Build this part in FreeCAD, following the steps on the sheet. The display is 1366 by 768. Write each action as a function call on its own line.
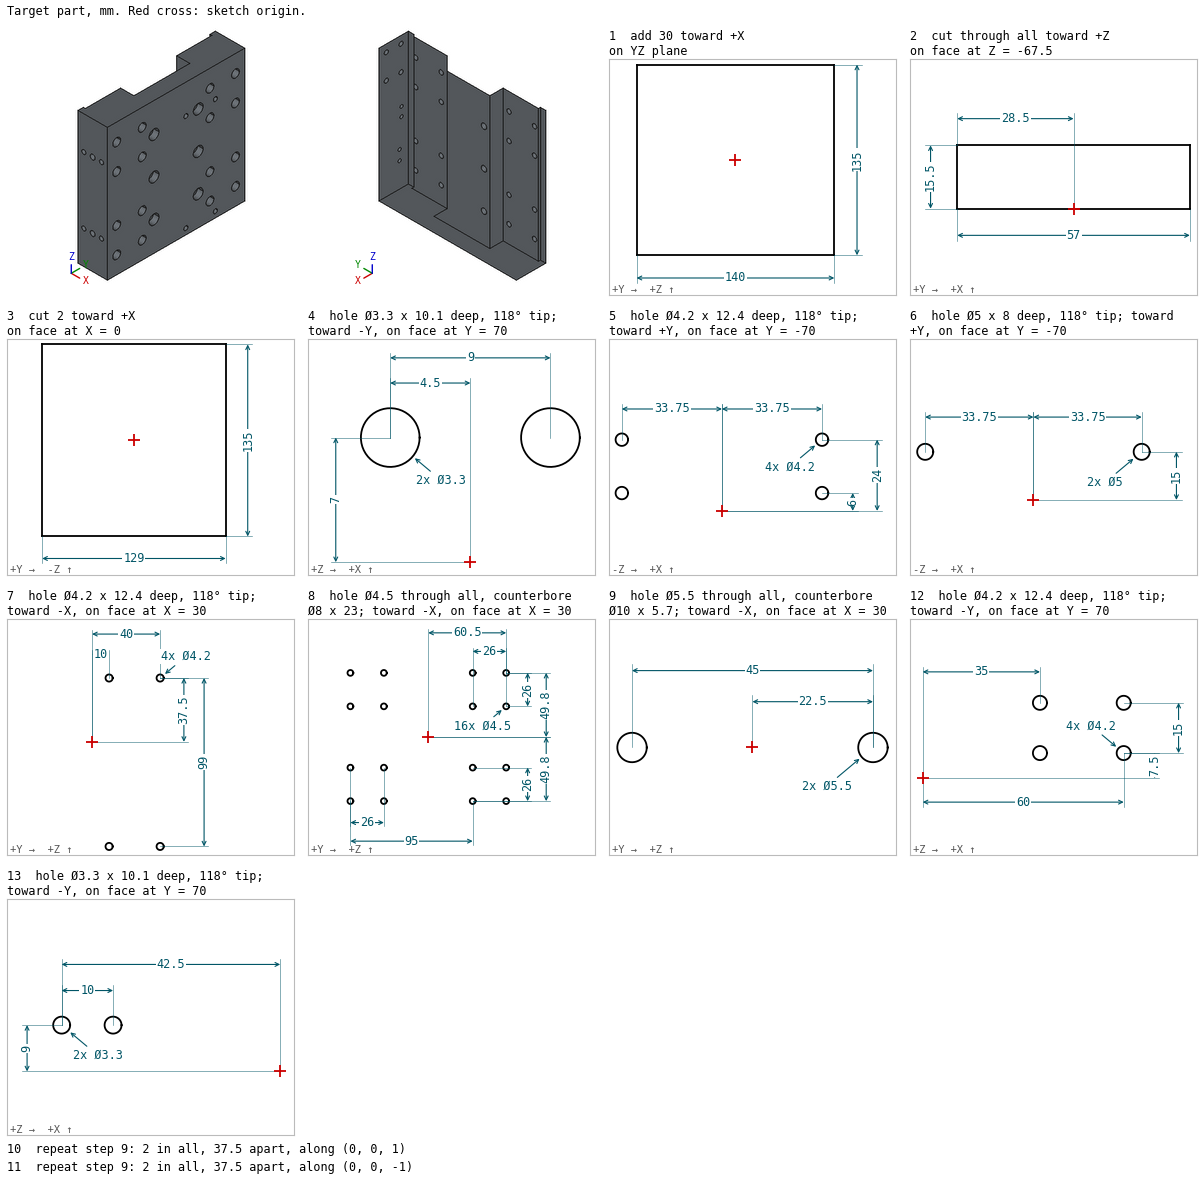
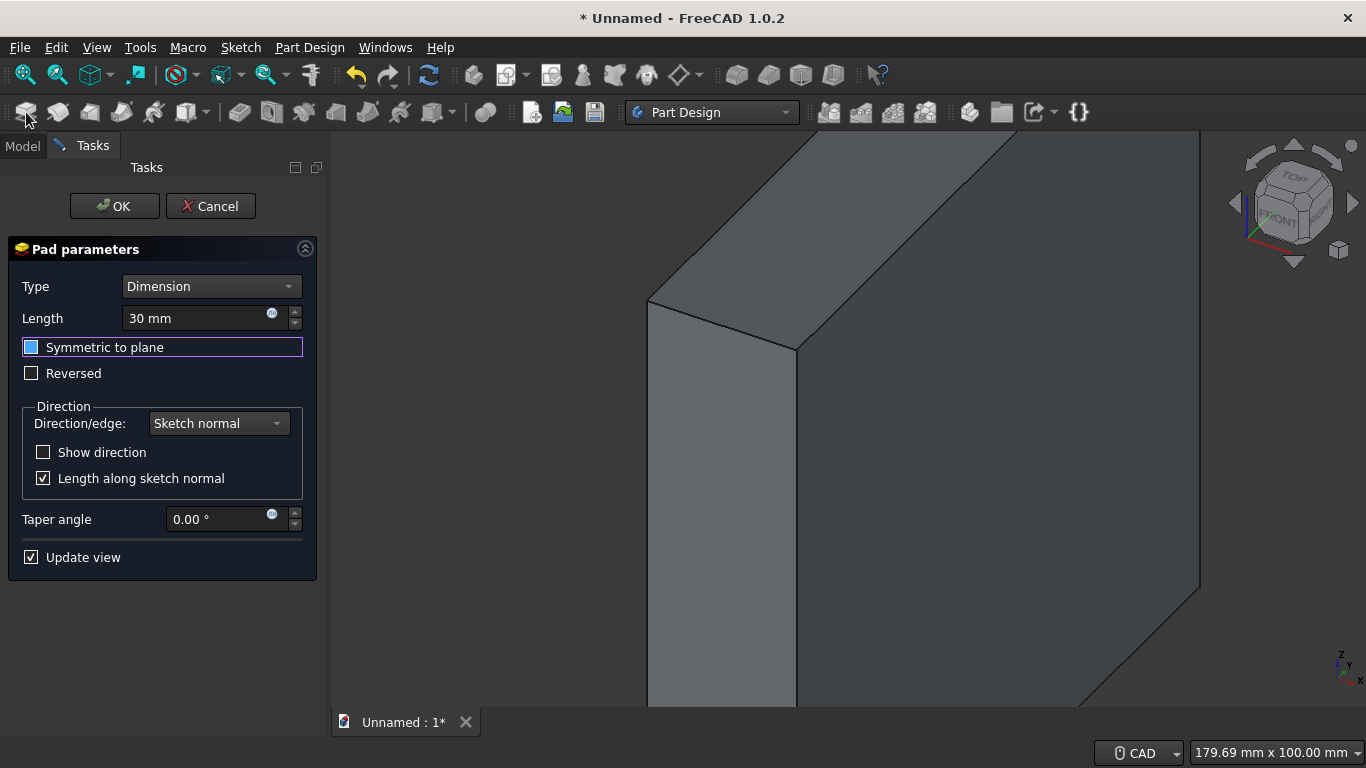
click(115, 206)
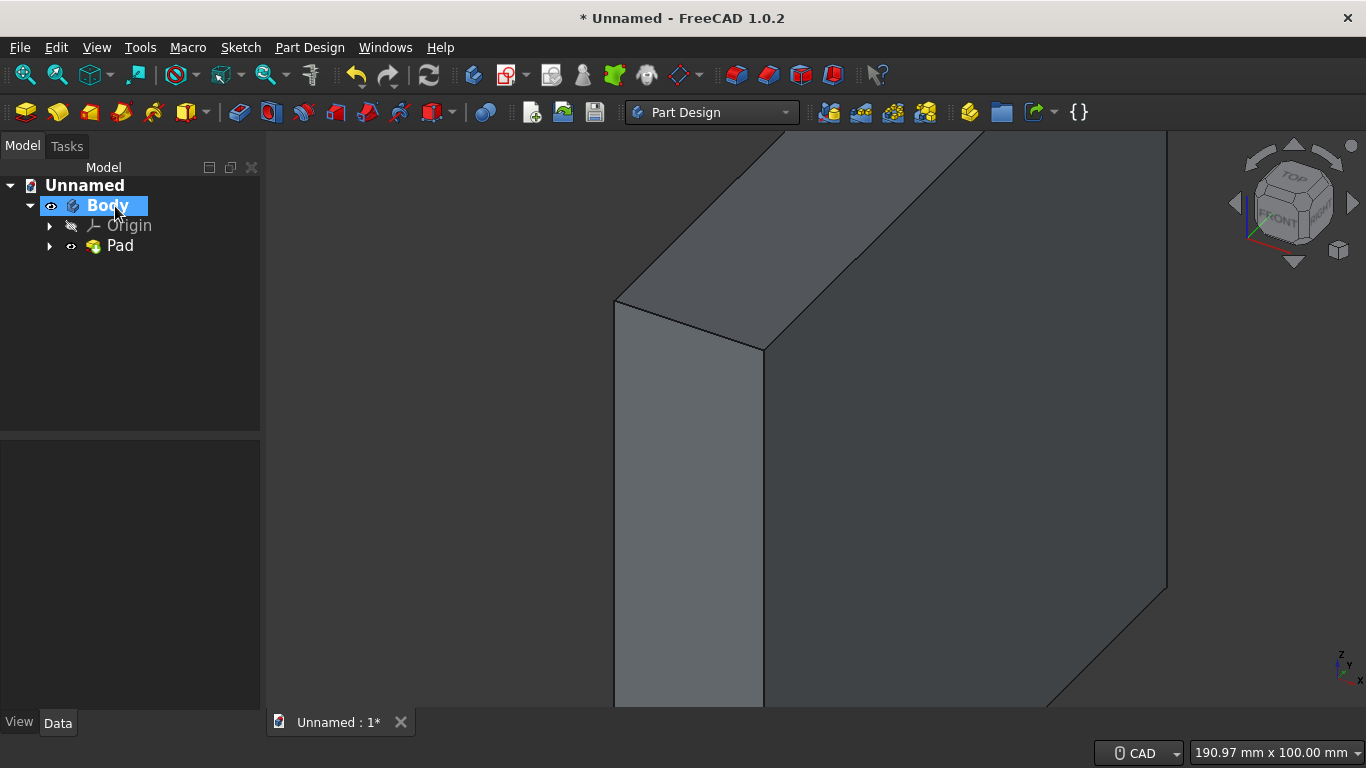
click(26, 76)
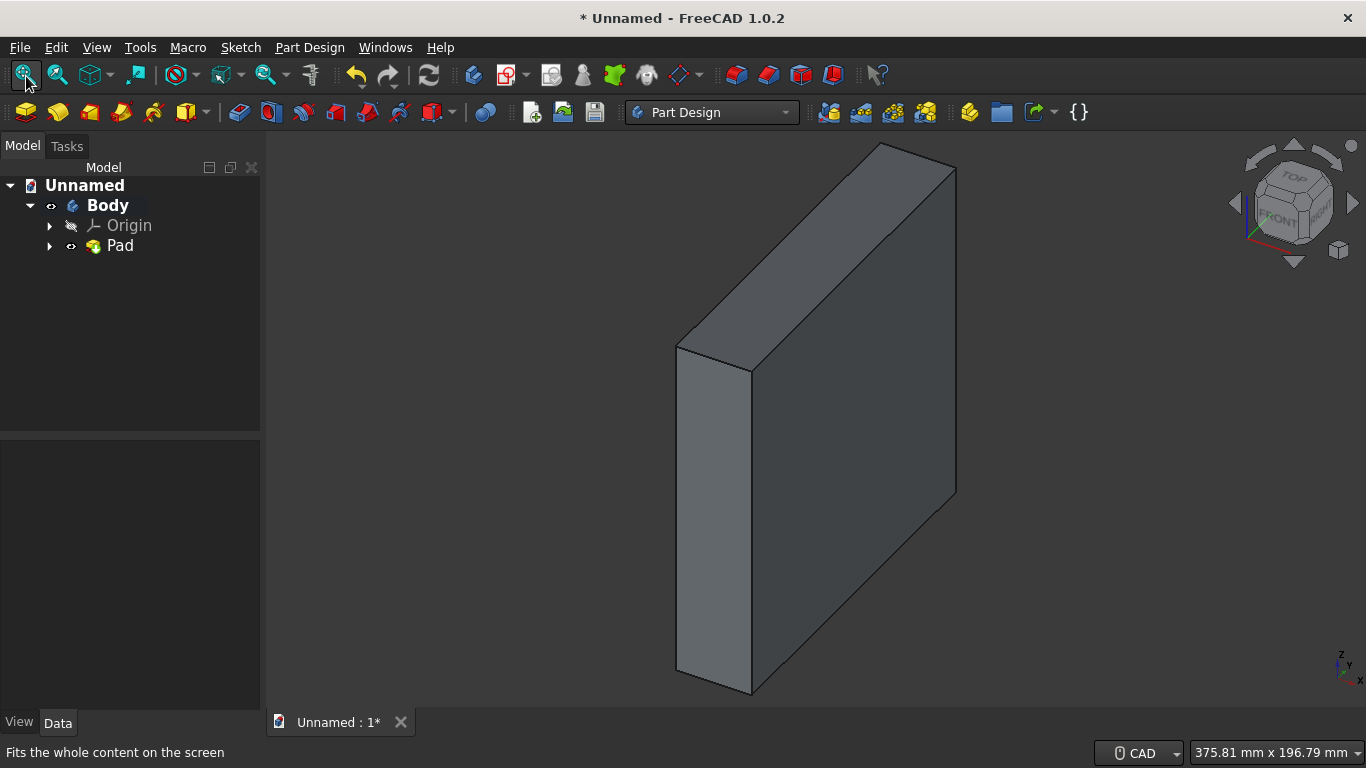
key(5)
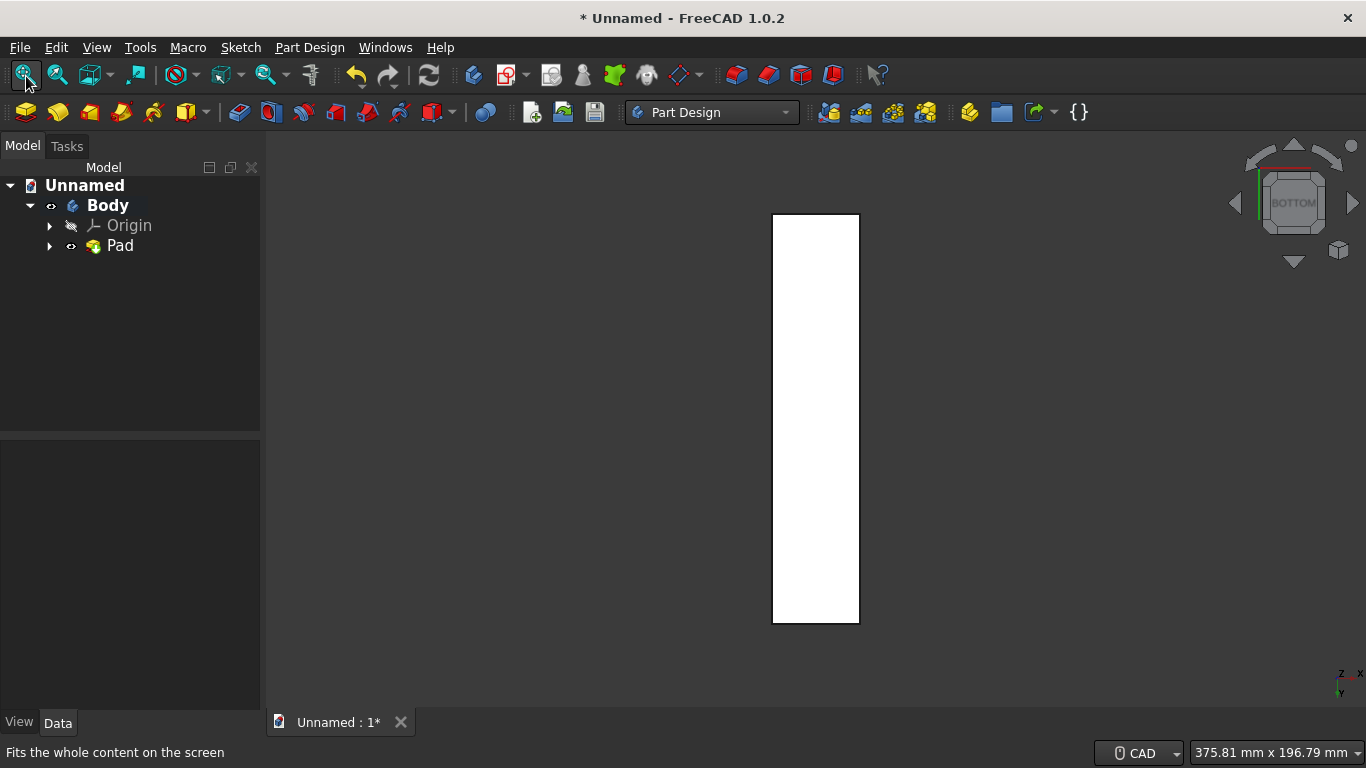
click(816, 535)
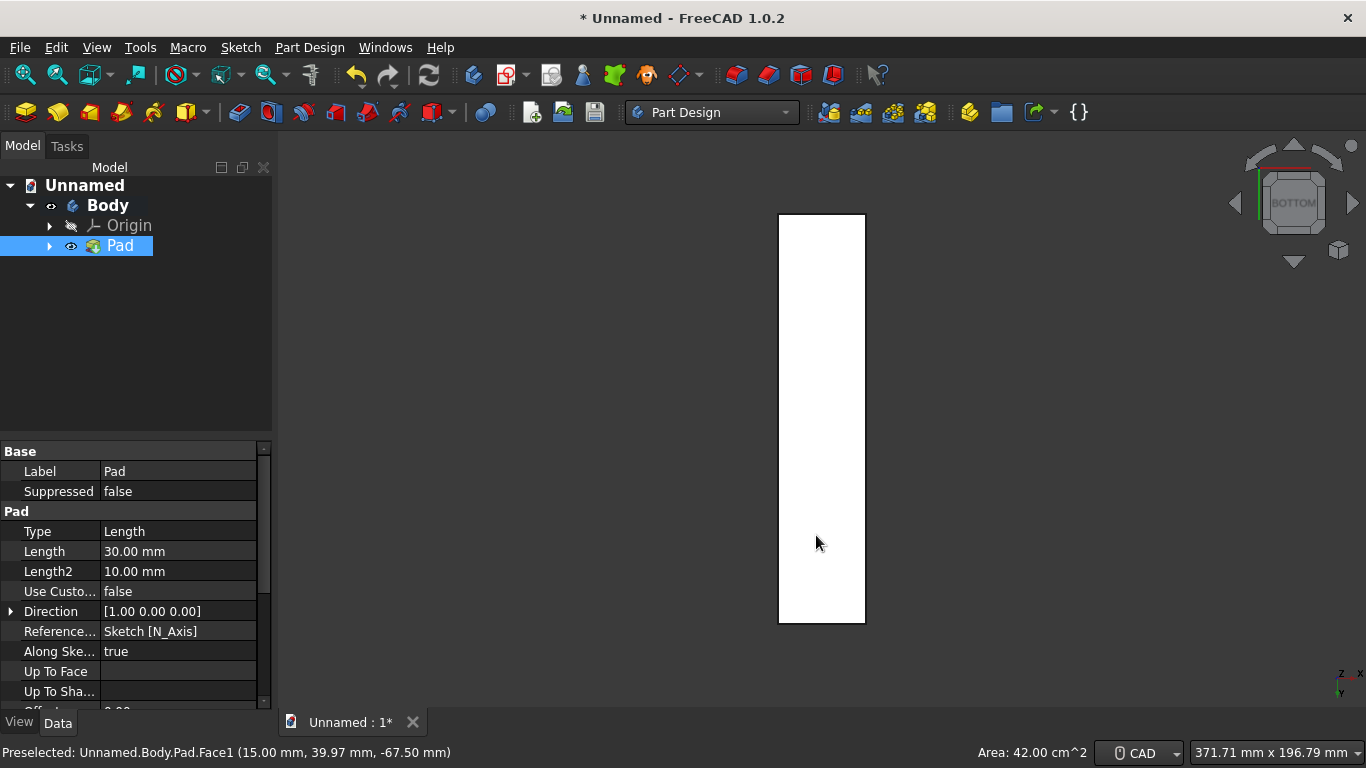
click(506, 76)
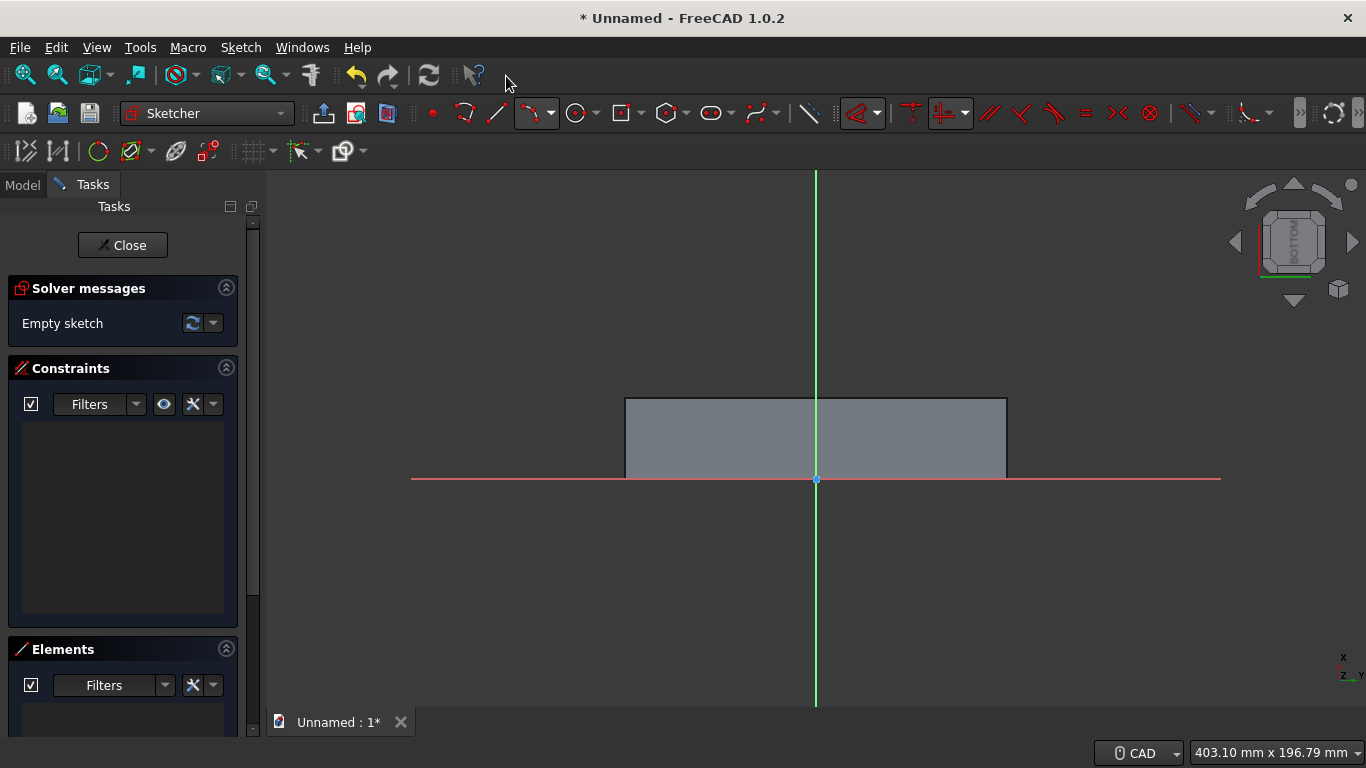
scroll(838, 465, up, 7)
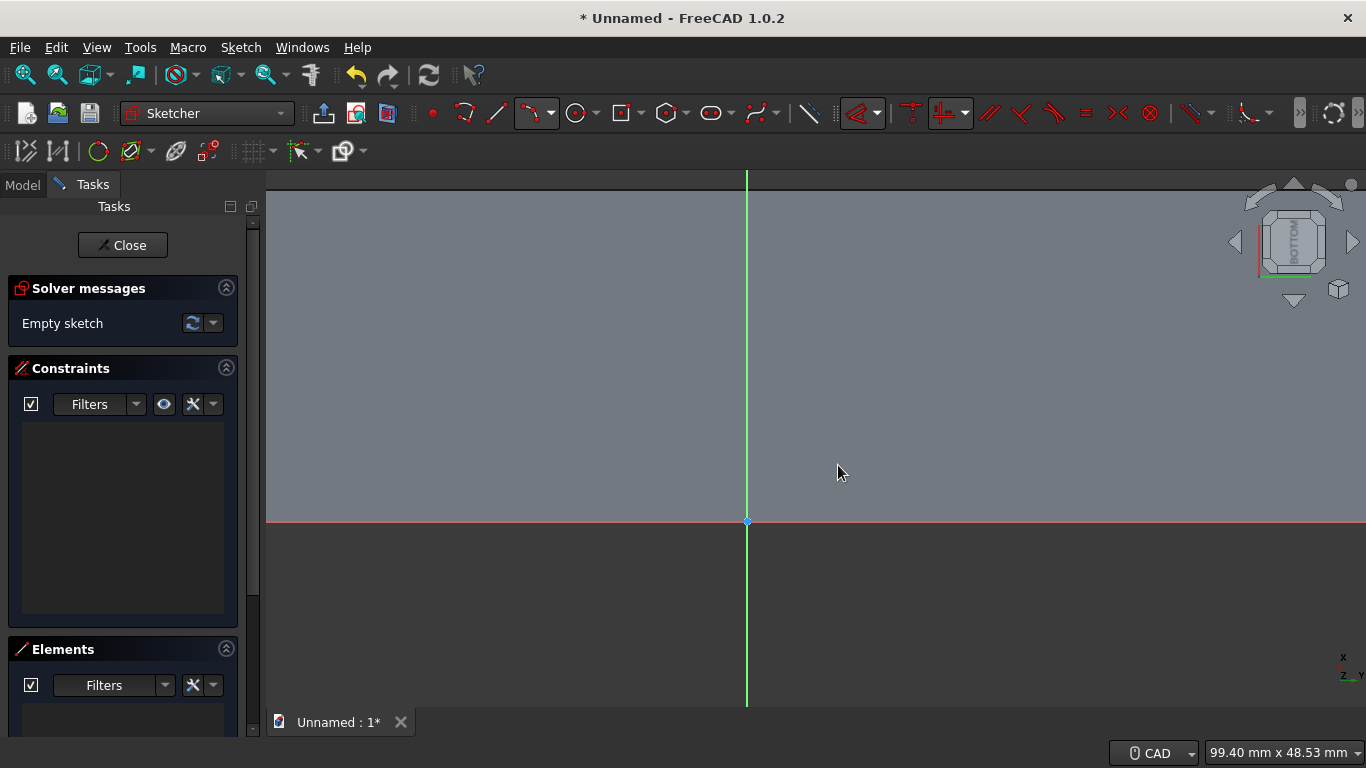
key(g)
key(r)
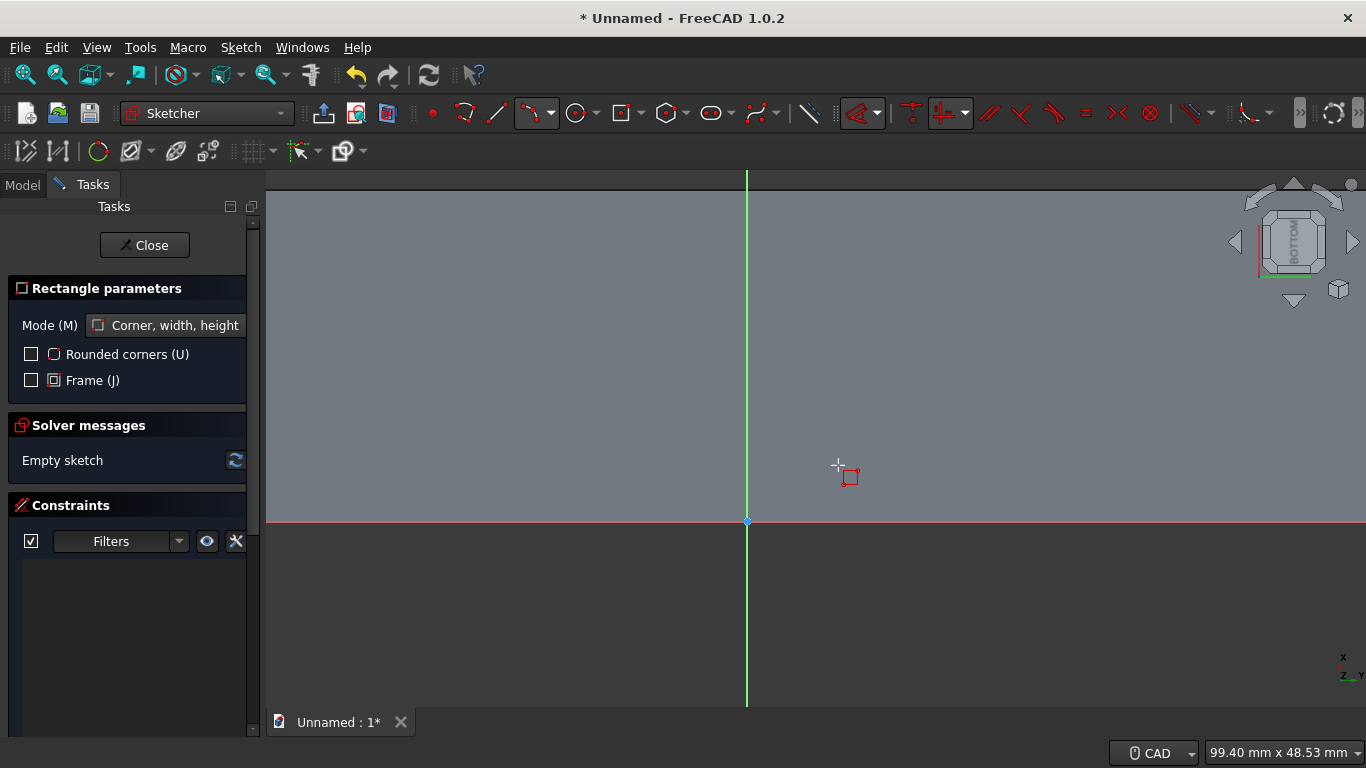
click(432, 350)
click(1063, 522)
key(Escape)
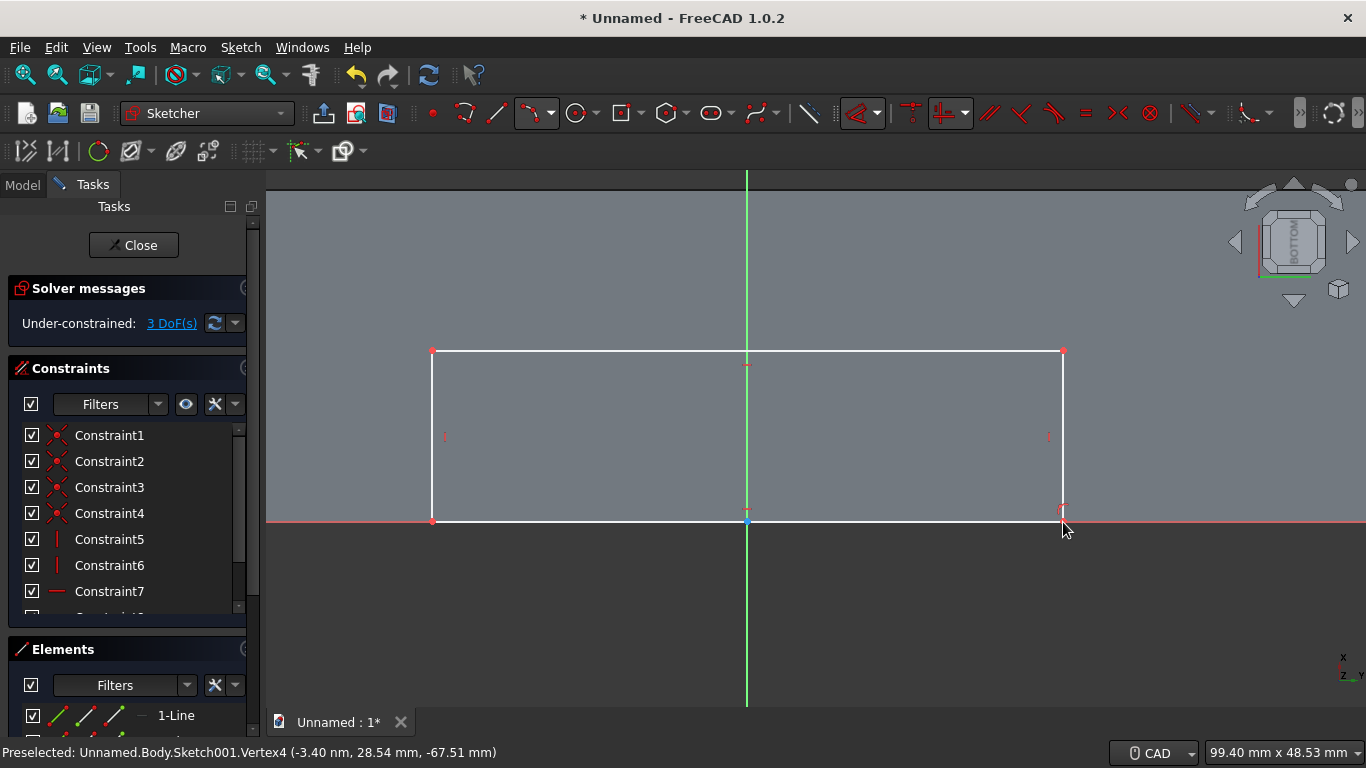
click(621, 522)